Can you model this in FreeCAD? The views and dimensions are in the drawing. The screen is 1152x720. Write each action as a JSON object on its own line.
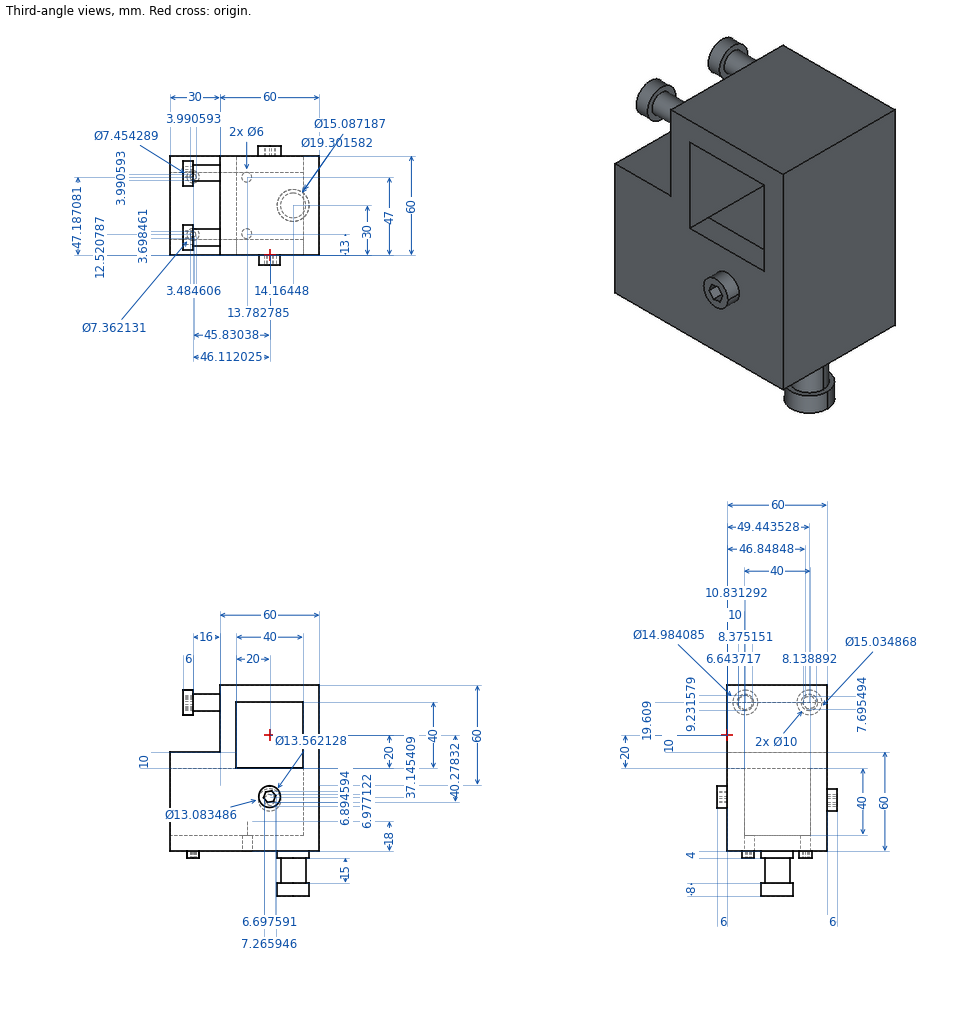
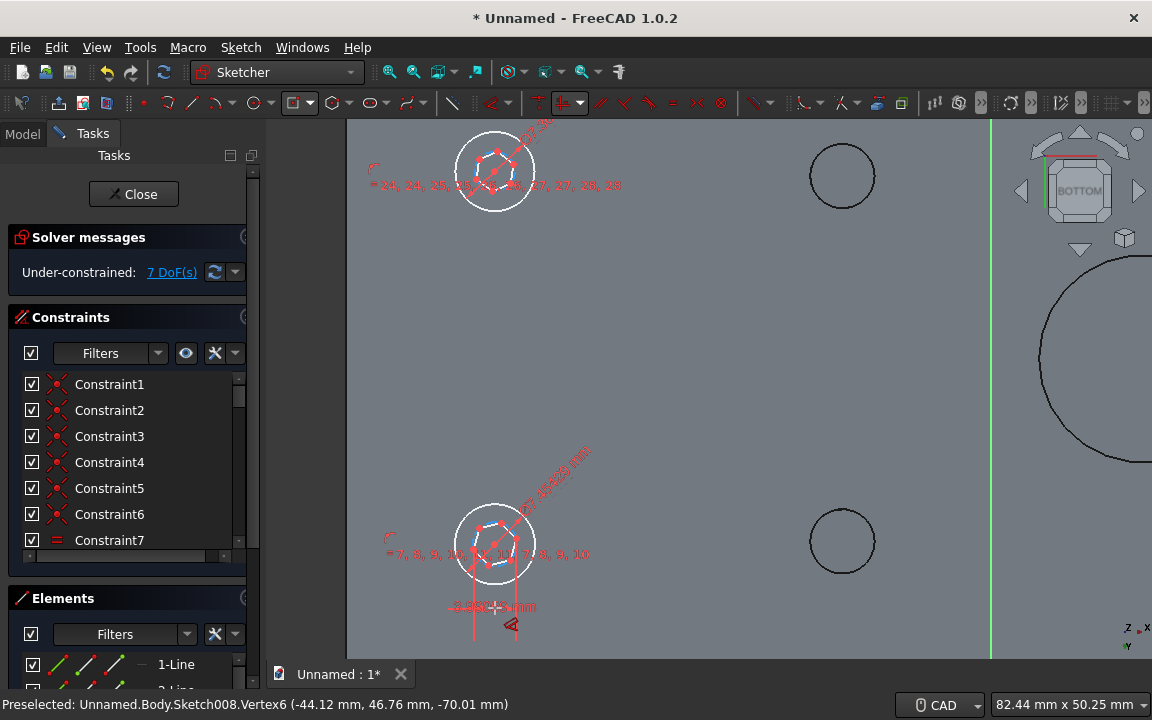
{"action": "left_click", "coordinate": [489, 566]}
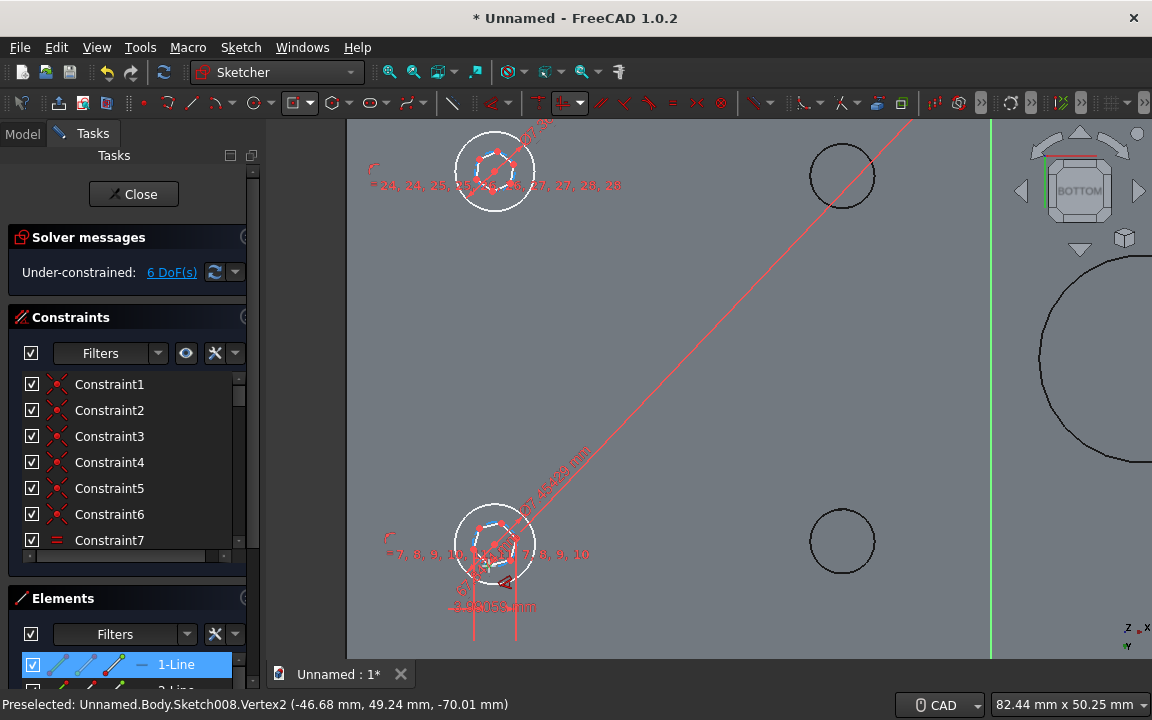
{"action": "left_click", "coordinate": [501, 523]}
{"action": "left_click", "coordinate": [431, 544]}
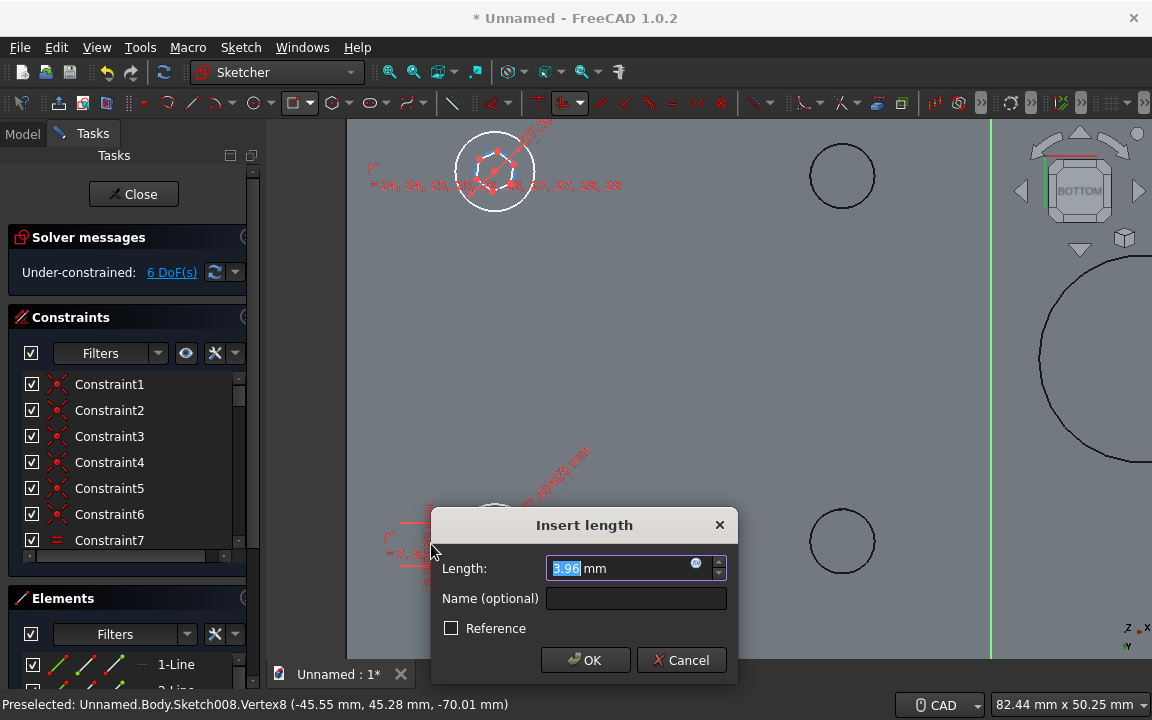
{"action": "type", "text": "3.990593"}
{"action": "key", "text": "Return"}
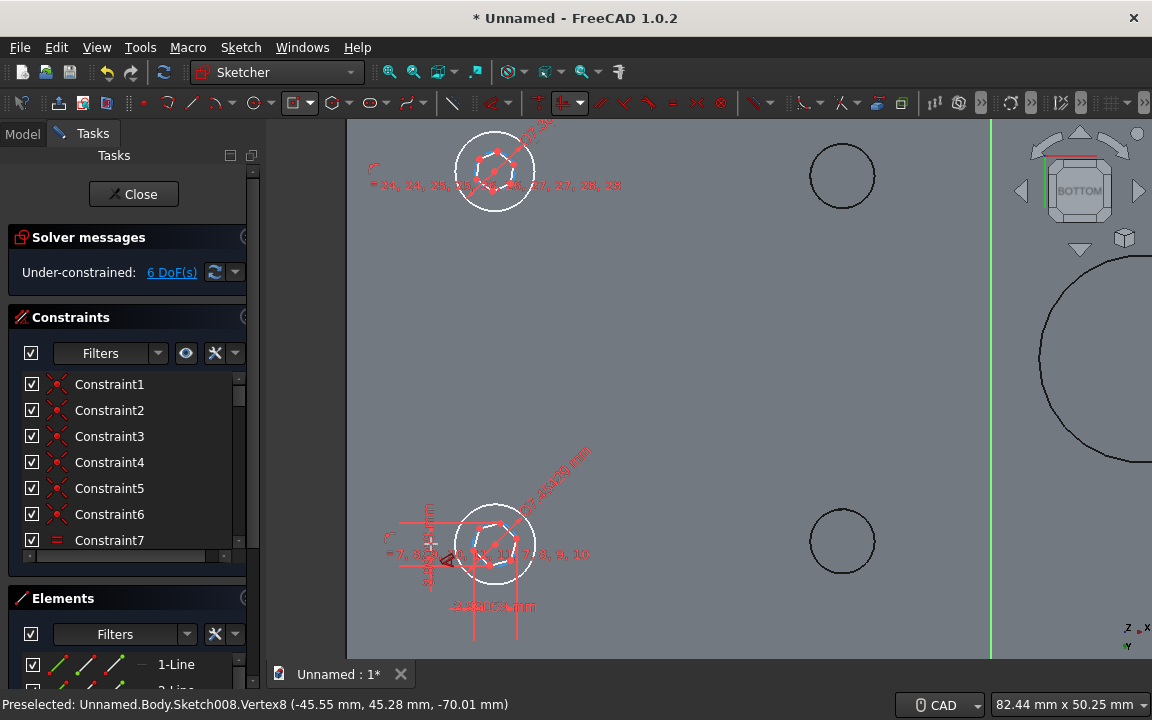
{"action": "left_click", "coordinate": [476, 179]}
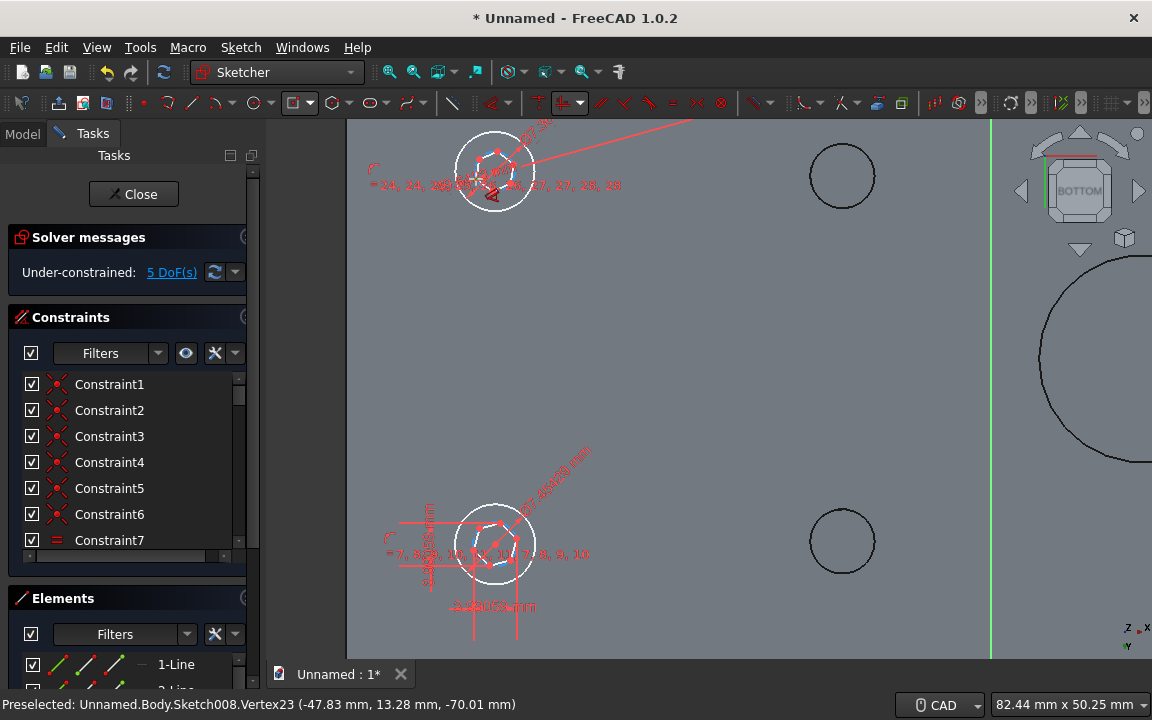
{"action": "left_click", "coordinate": [513, 164]}
{"action": "left_click", "coordinate": [495, 237]}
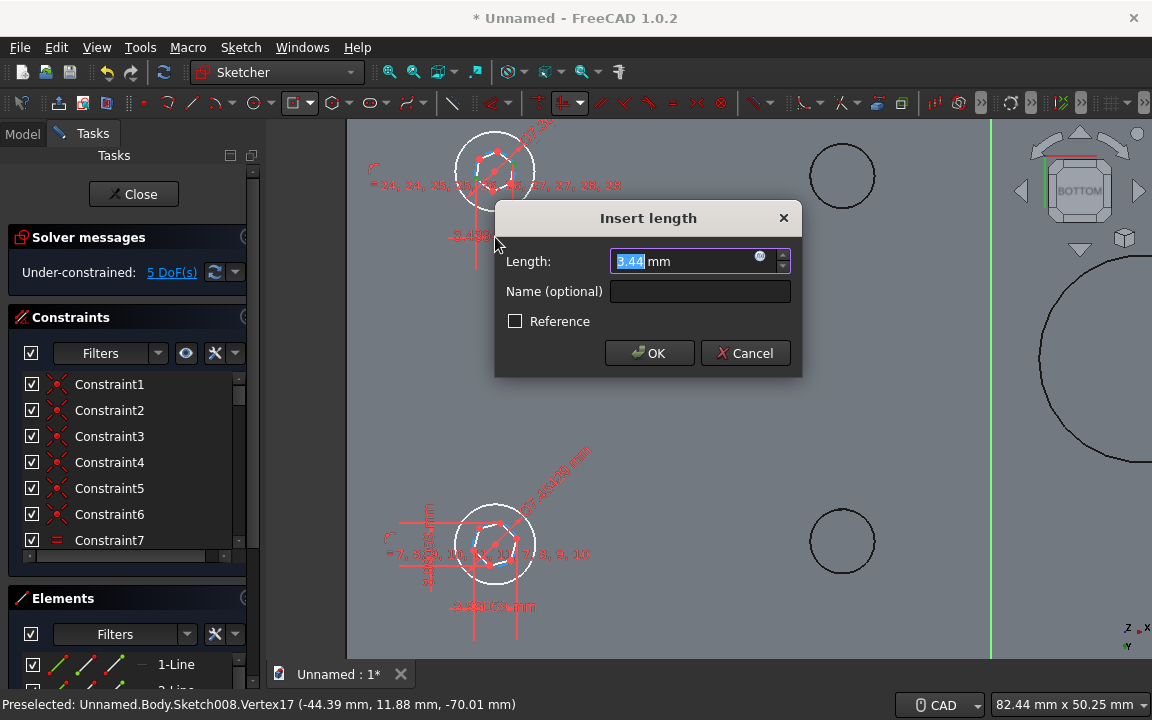
{"action": "type", "text": "3.484606"}
{"action": "key", "text": "Return"}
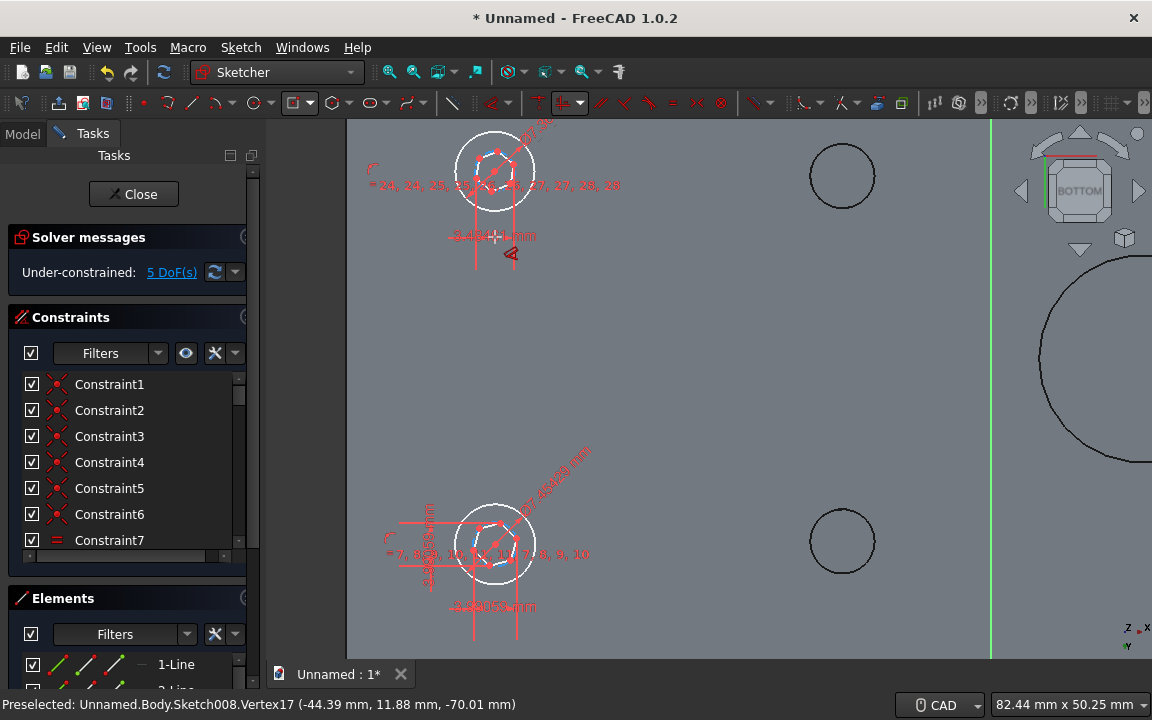
{"action": "left_click", "coordinate": [492, 191]}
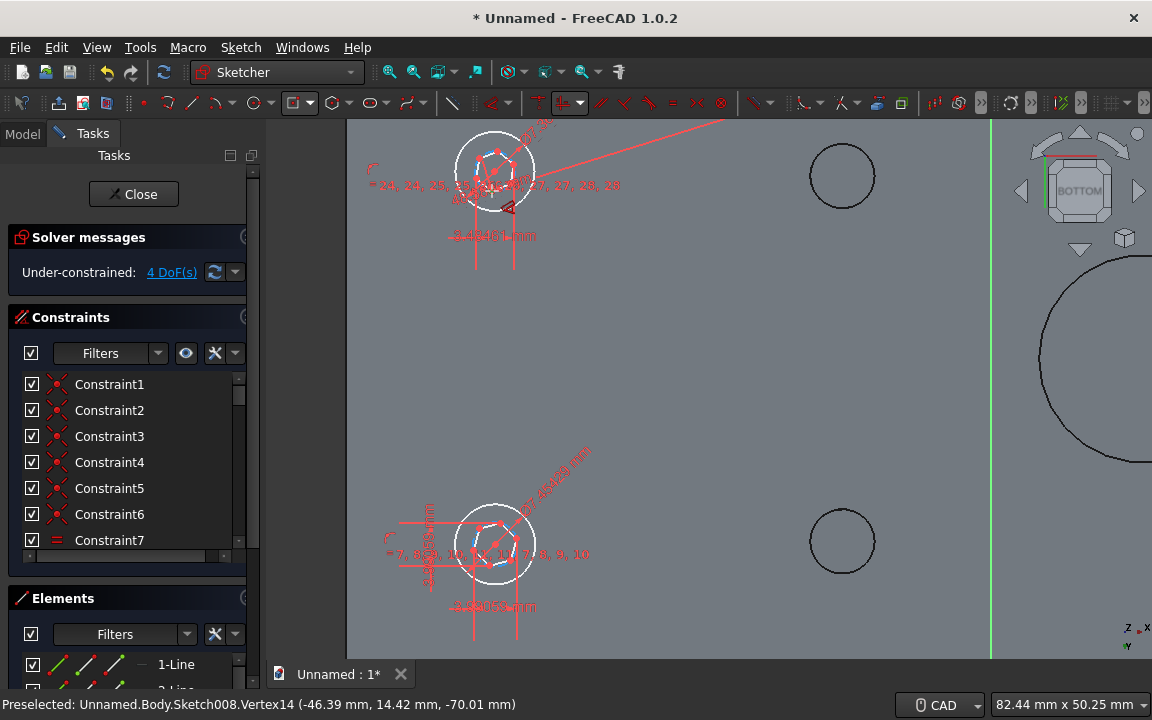
{"action": "left_click", "coordinate": [498, 152]}
{"action": "left_click", "coordinate": [434, 171]}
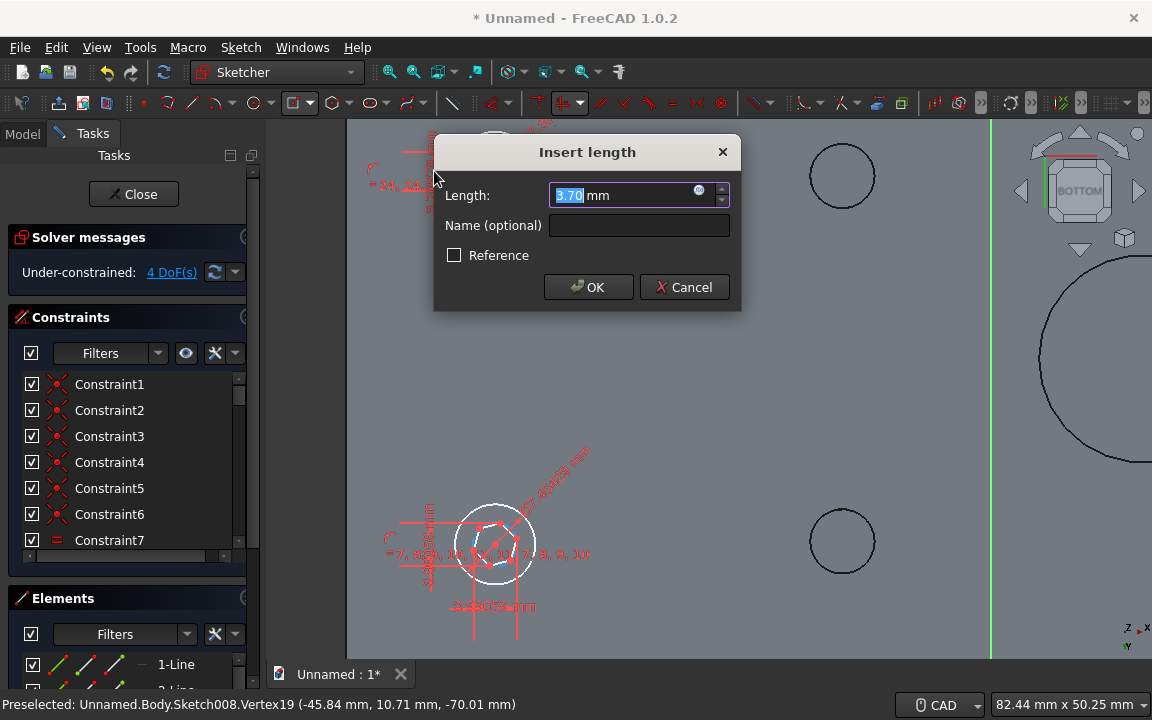
{"action": "type", "text": "3.698461"}
{"action": "key", "text": "Return"}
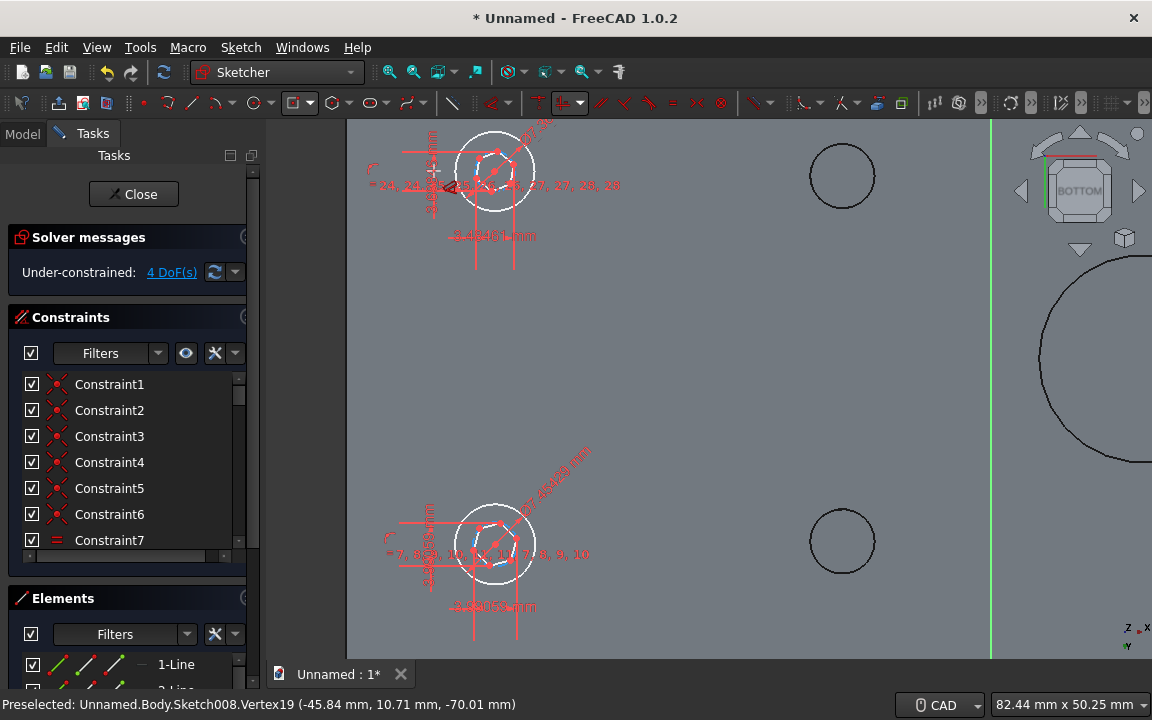
{"action": "left_click", "coordinate": [498, 152]}
{"action": "left_click", "coordinate": [742, 186]}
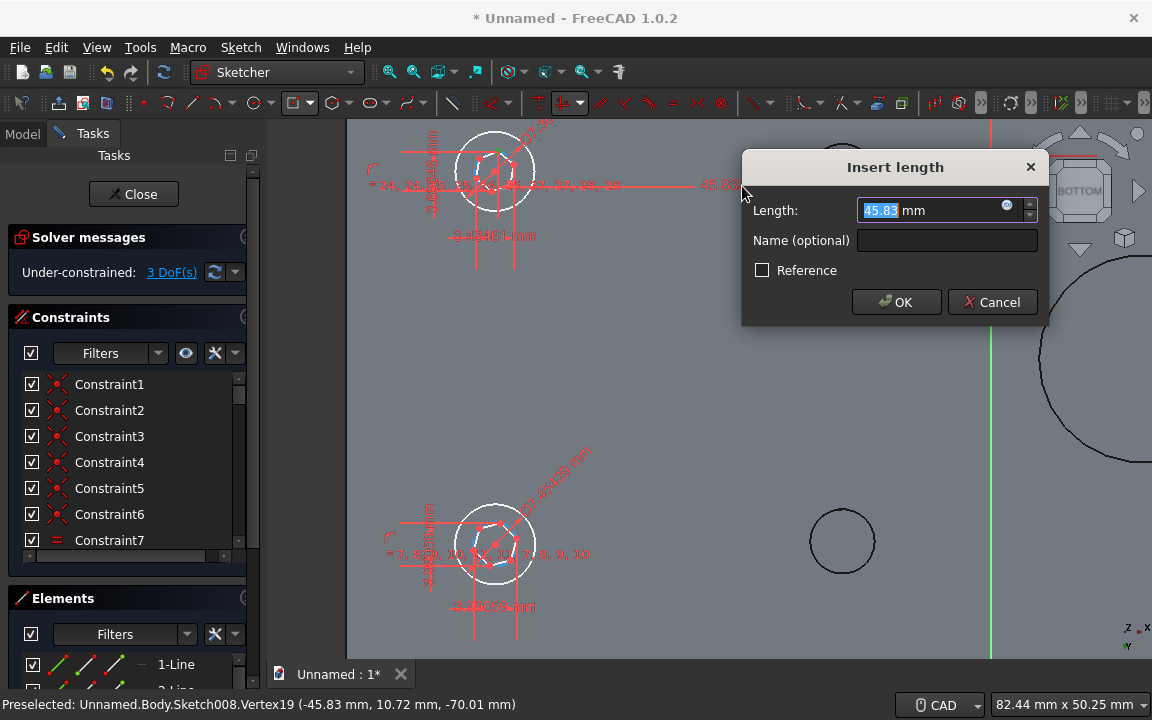
{"action": "type", "text": "45.83038"}
{"action": "key", "text": "Return"}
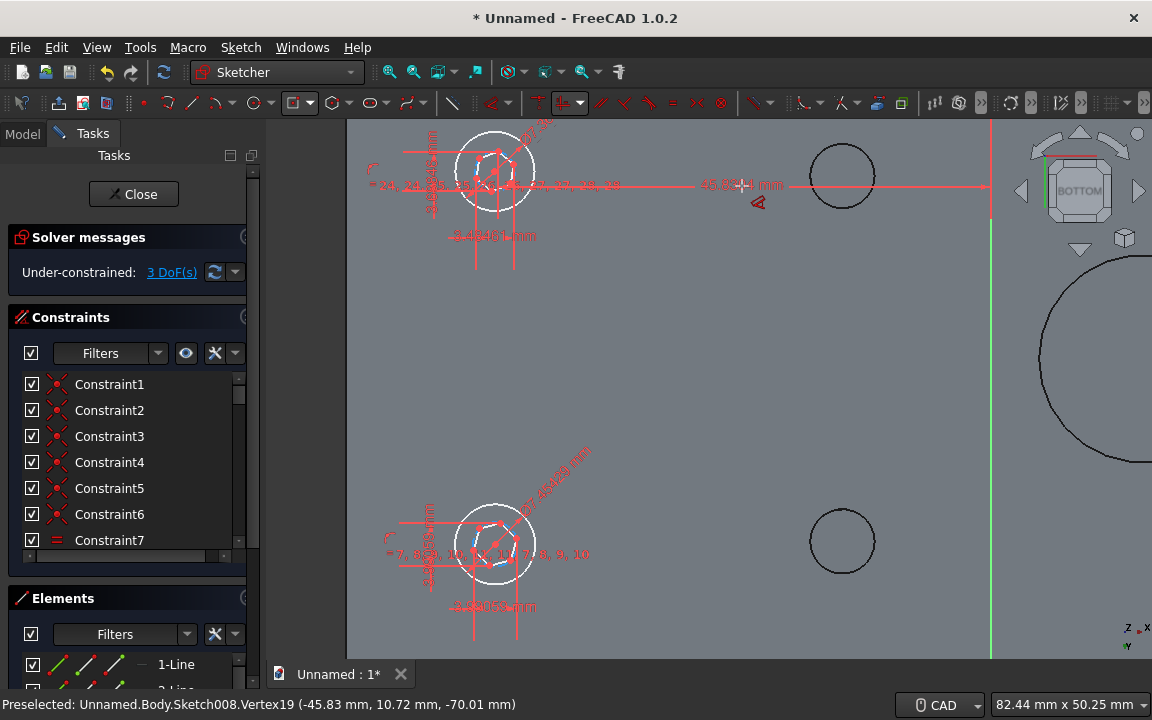
{"action": "left_click", "coordinate": [495, 544]}
{"action": "left_click", "coordinate": [741, 578]}